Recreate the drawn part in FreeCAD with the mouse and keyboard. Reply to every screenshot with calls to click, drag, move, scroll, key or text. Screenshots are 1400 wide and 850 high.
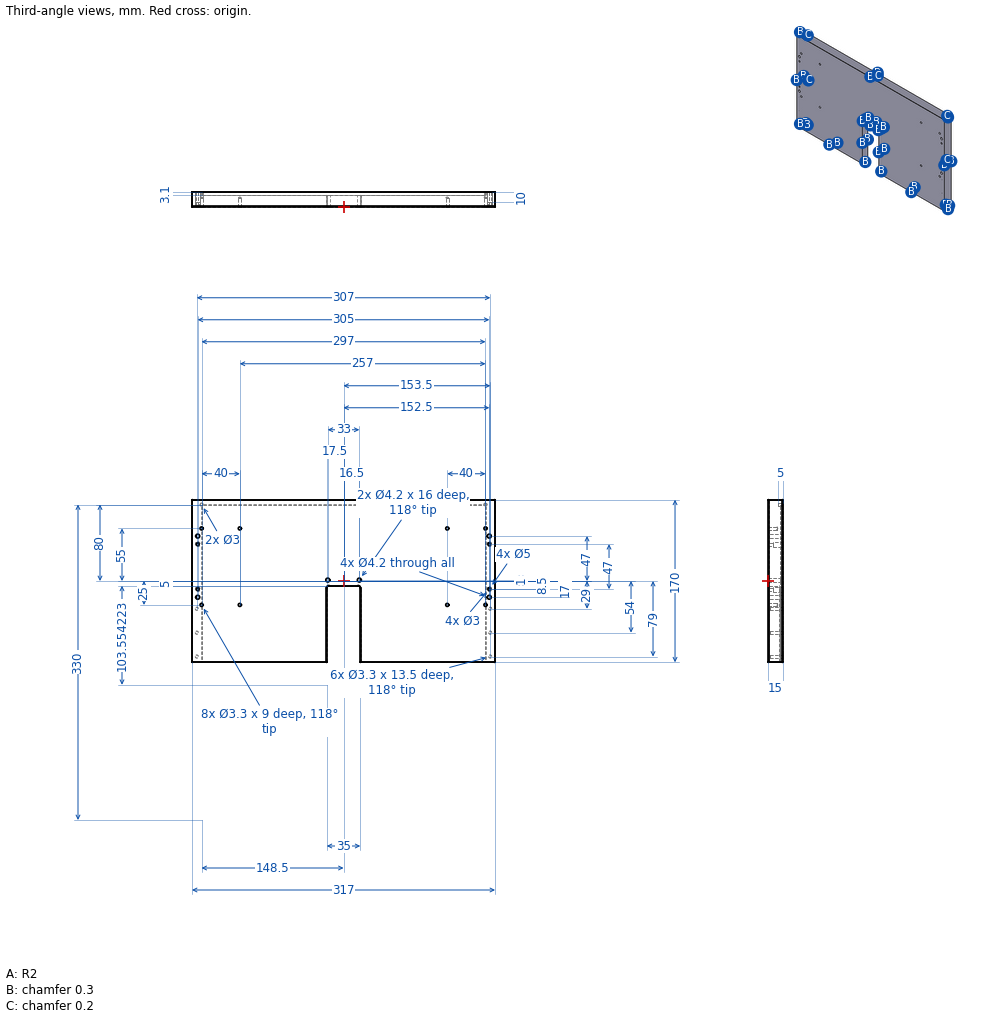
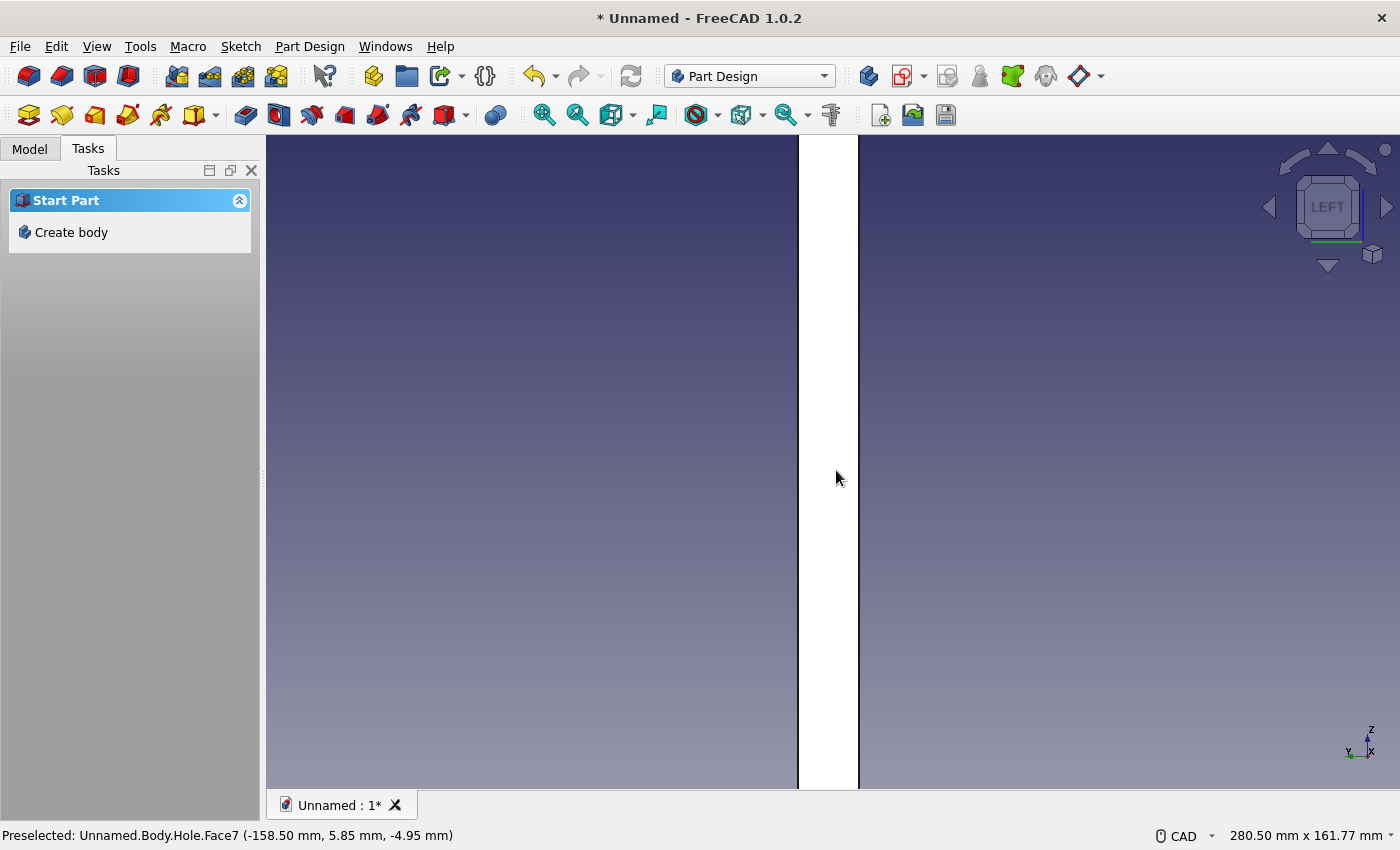
key(v)
key(f)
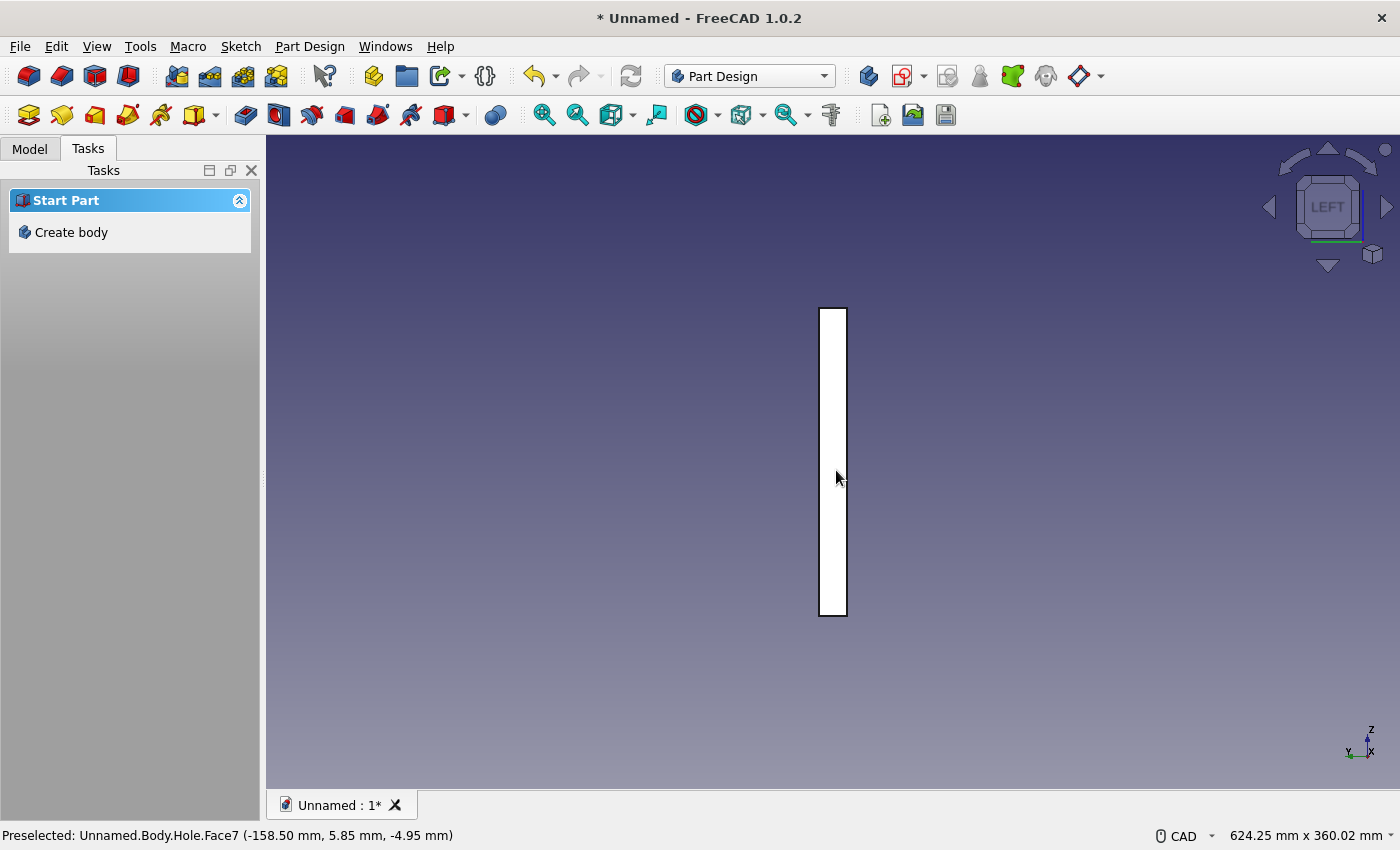
key(v)
key(3)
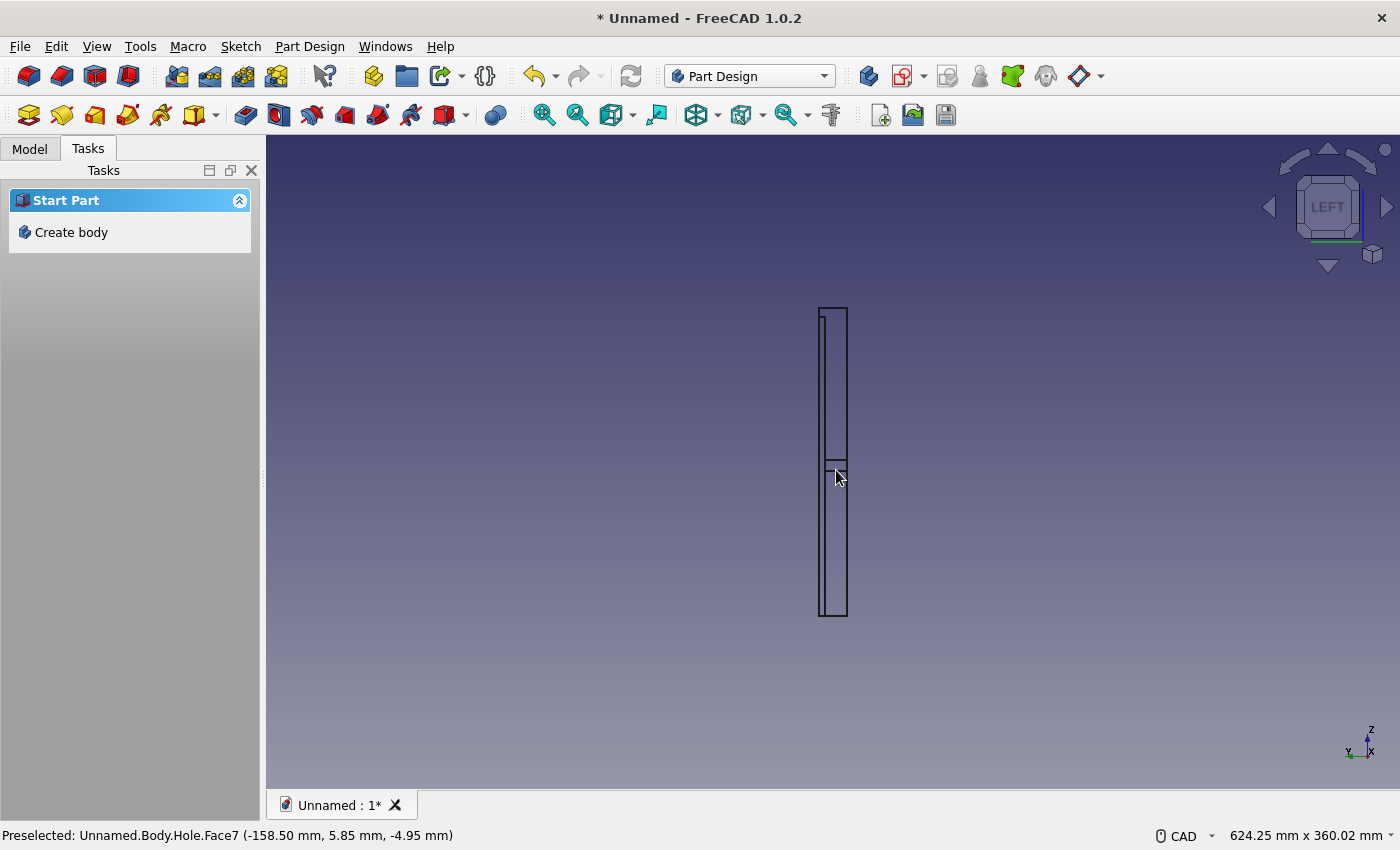
key(0)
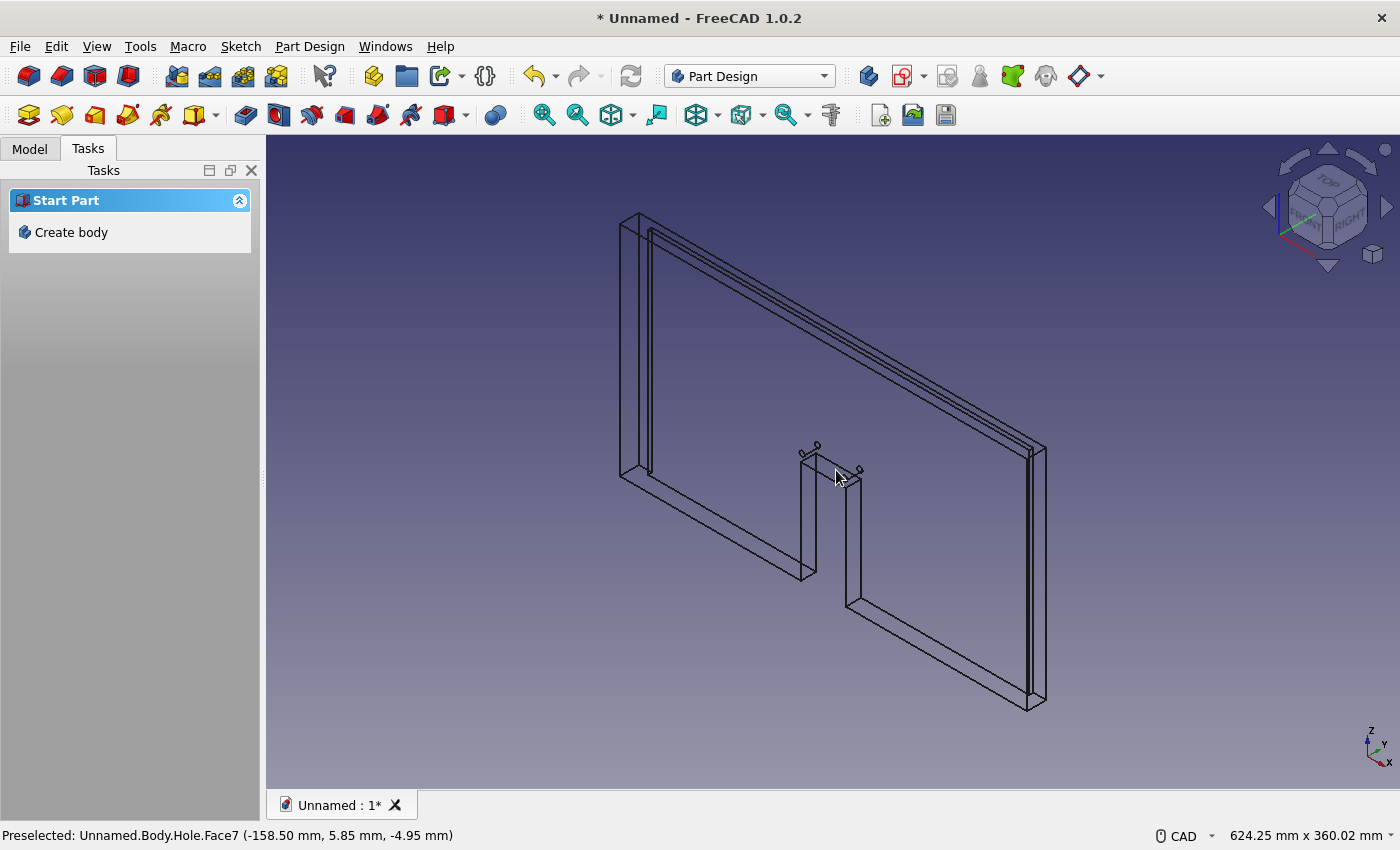
click(853, 483)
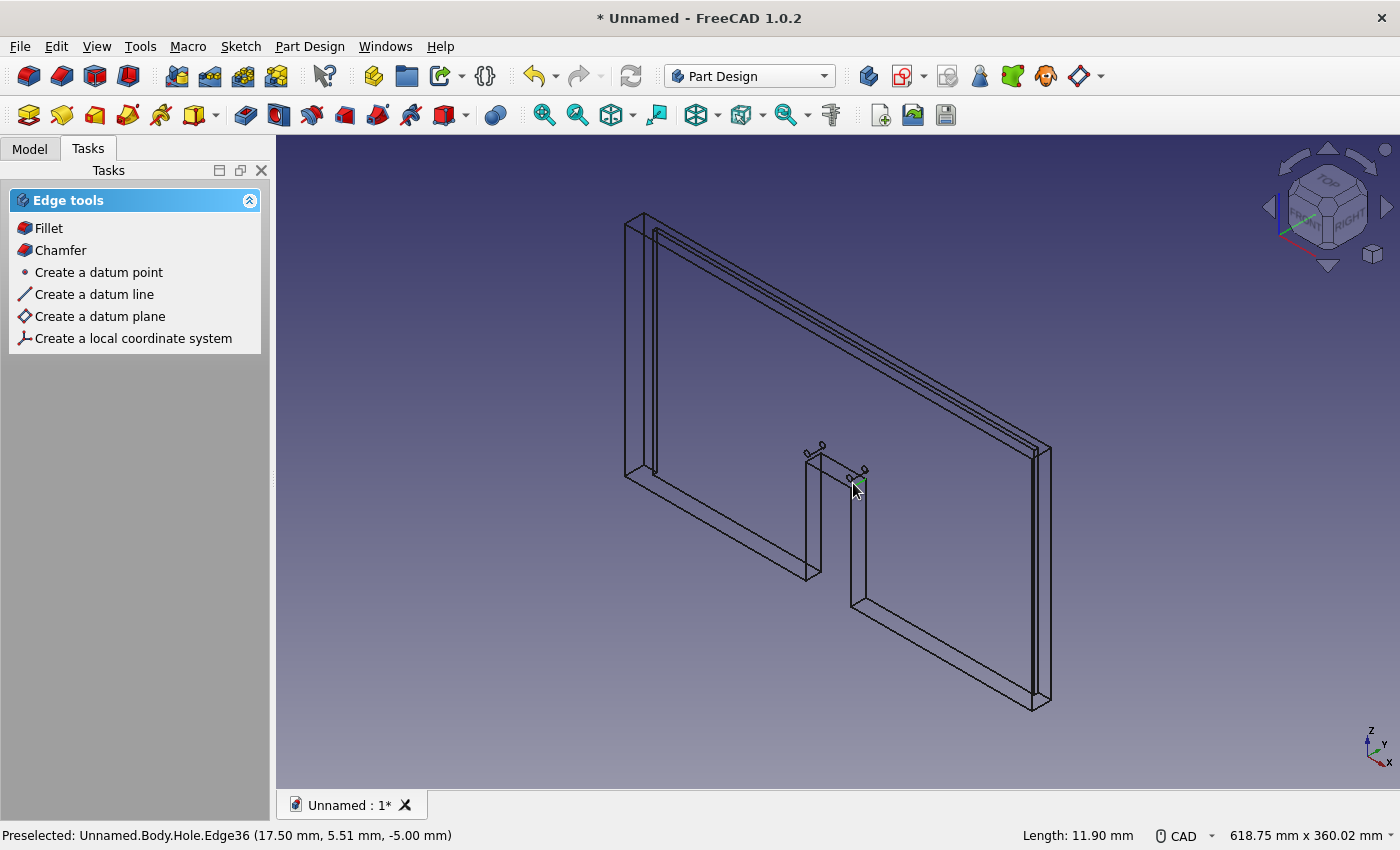
scroll(814, 457, up, 6)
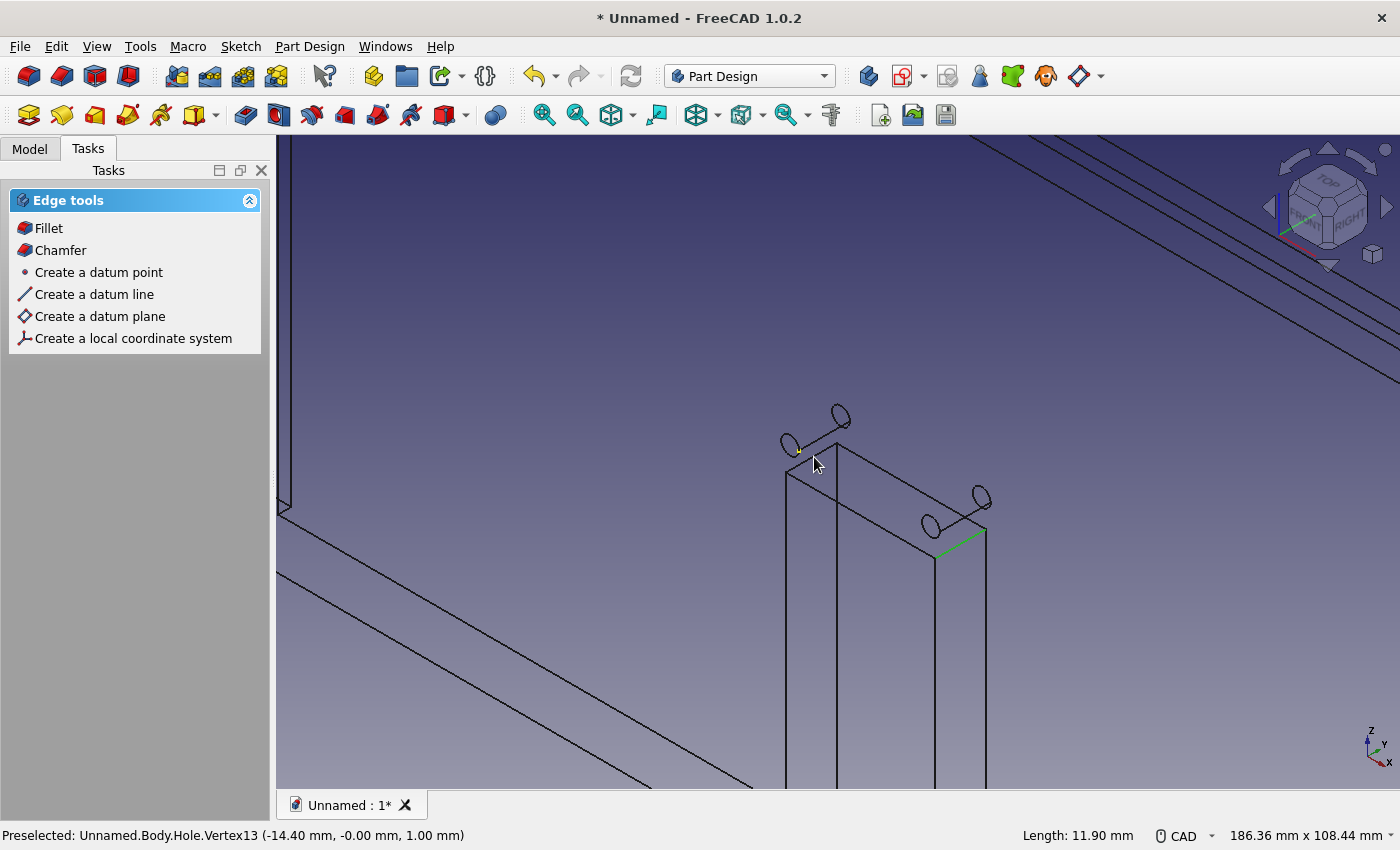
click(811, 457, ctrl)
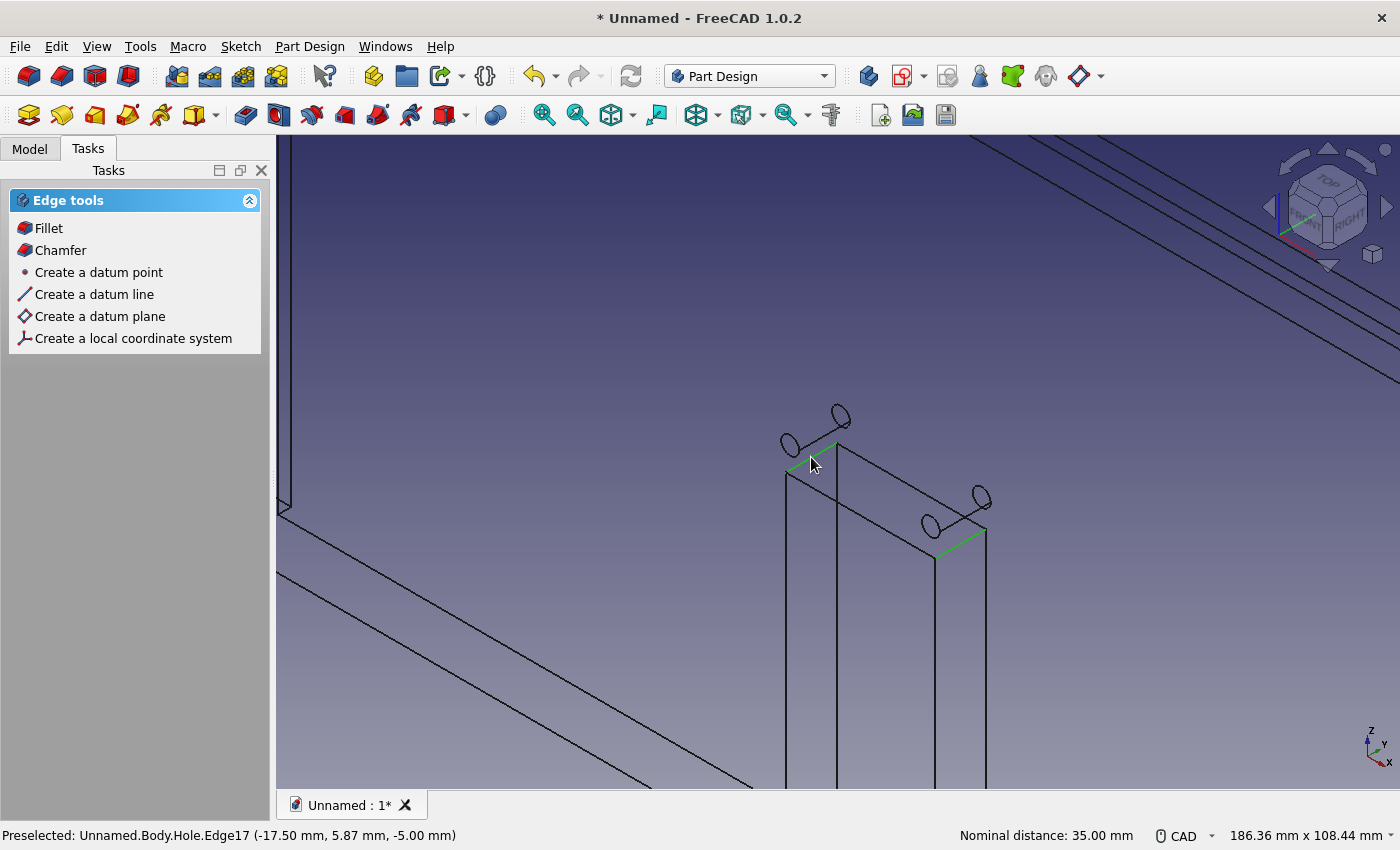
key(v)
key(1)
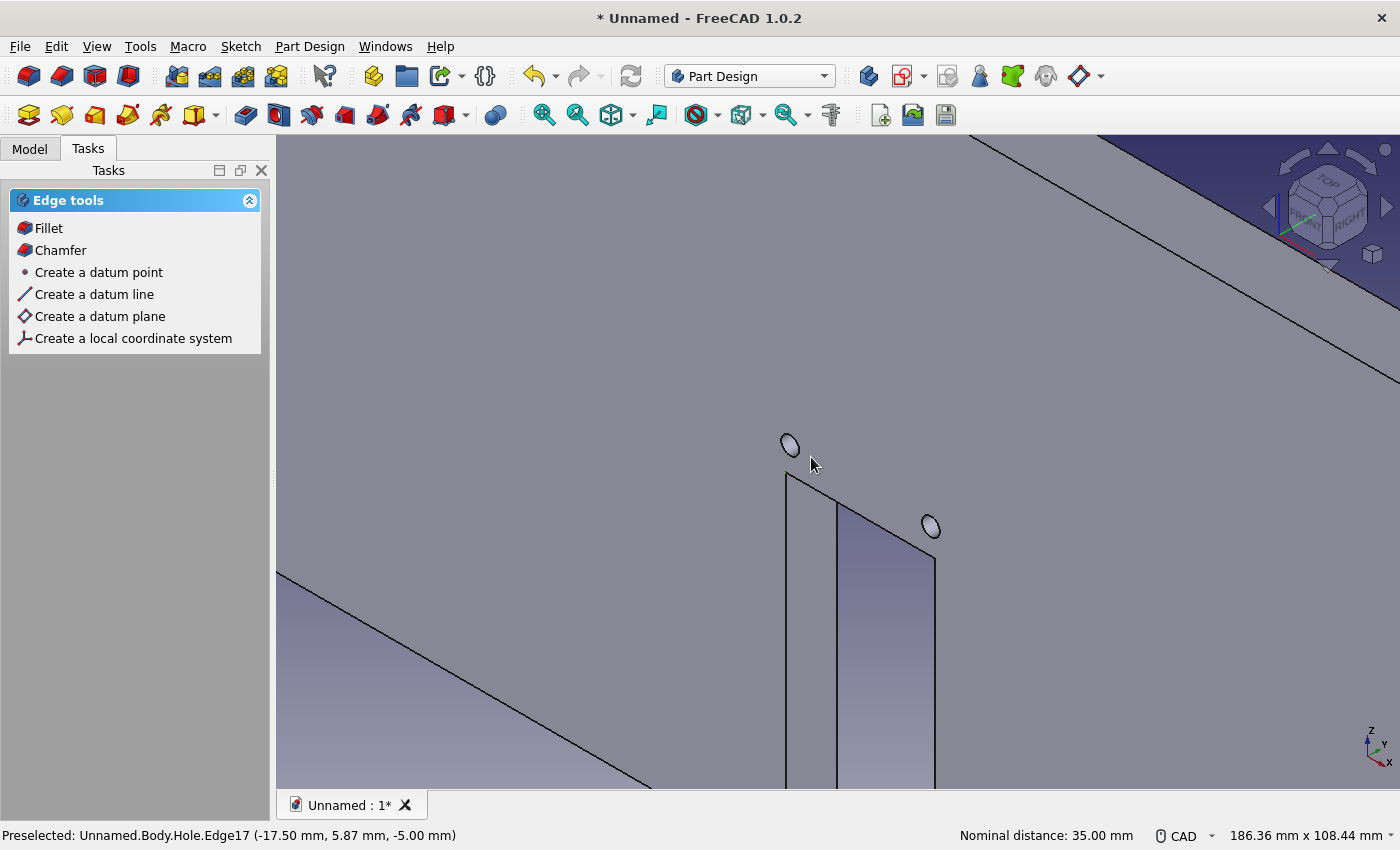
click(29, 76)